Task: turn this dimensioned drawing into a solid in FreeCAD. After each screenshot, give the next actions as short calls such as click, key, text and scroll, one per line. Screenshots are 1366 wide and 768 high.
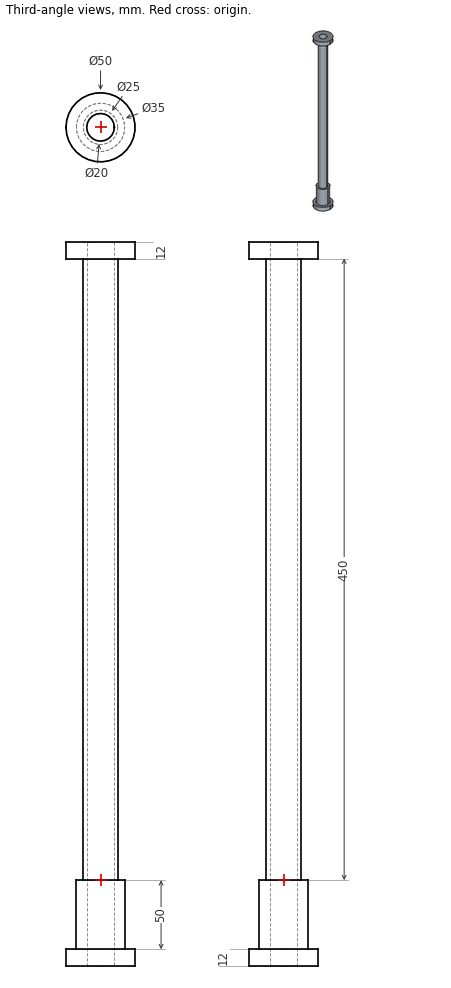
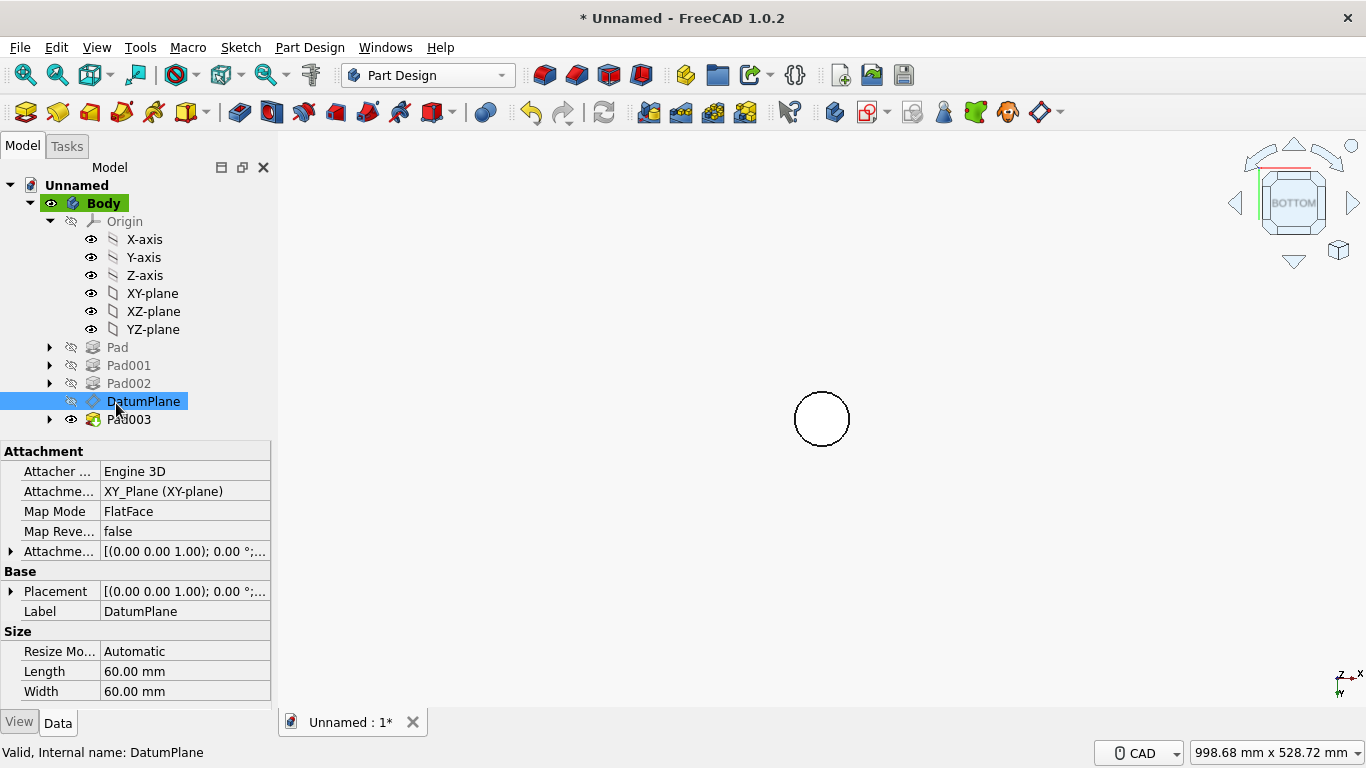
key(0)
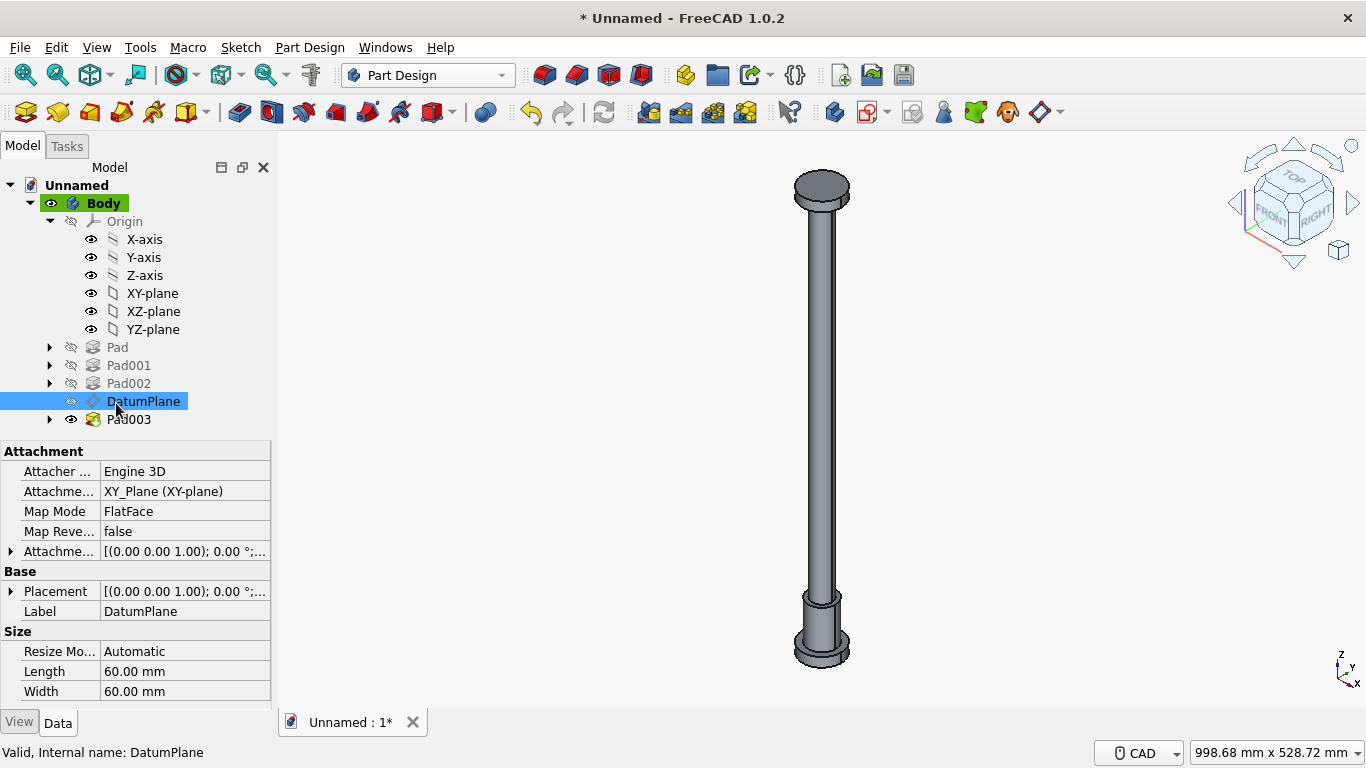
click(822, 185)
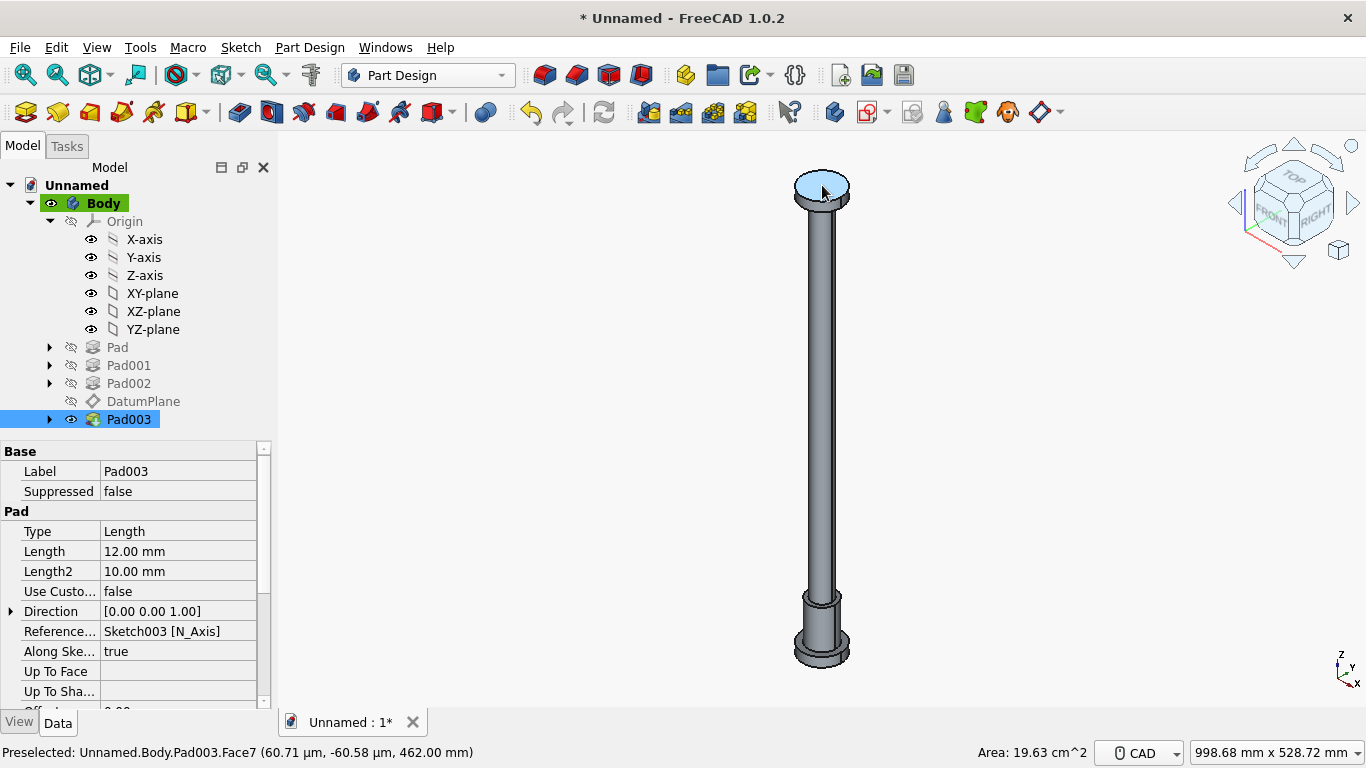
click(868, 112)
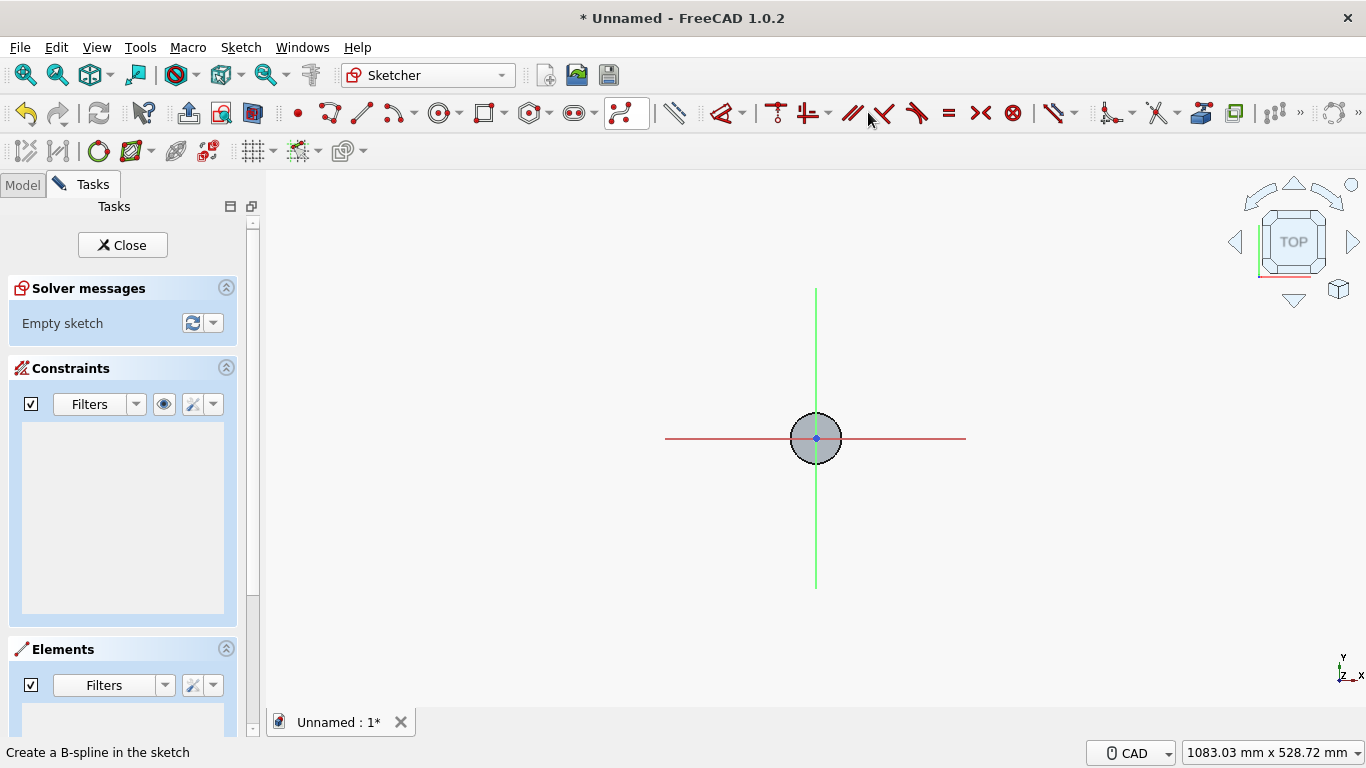
scroll(820, 438, up, 14)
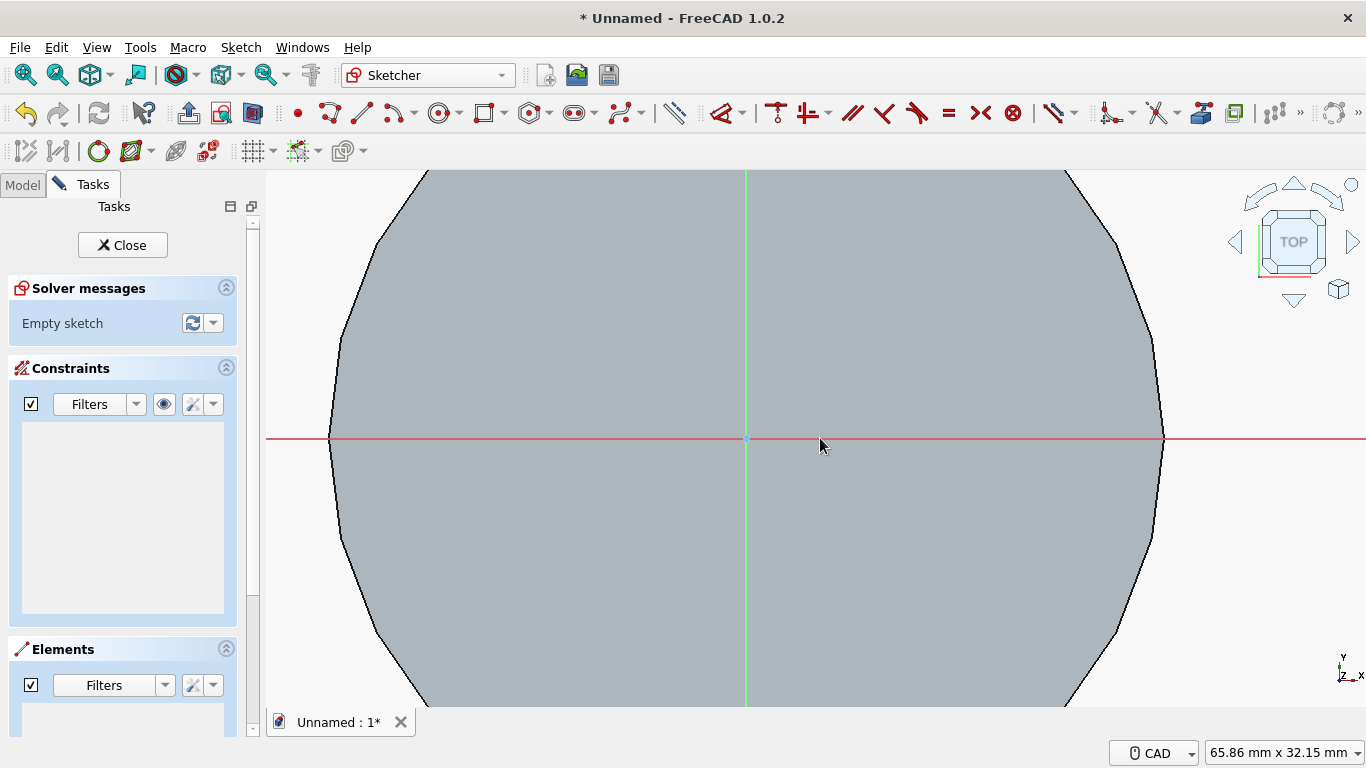
key(g)
key(c)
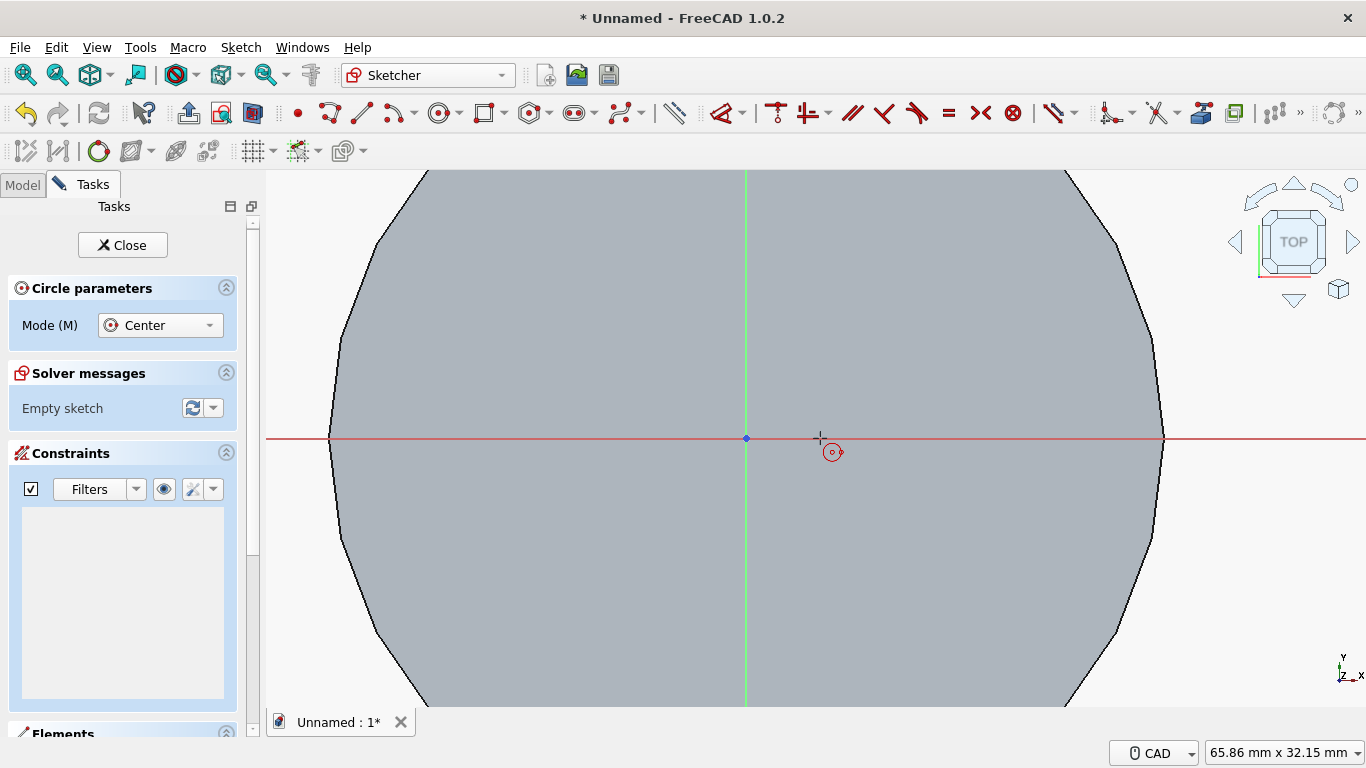
click(746, 438)
click(865, 320)
key(Escape)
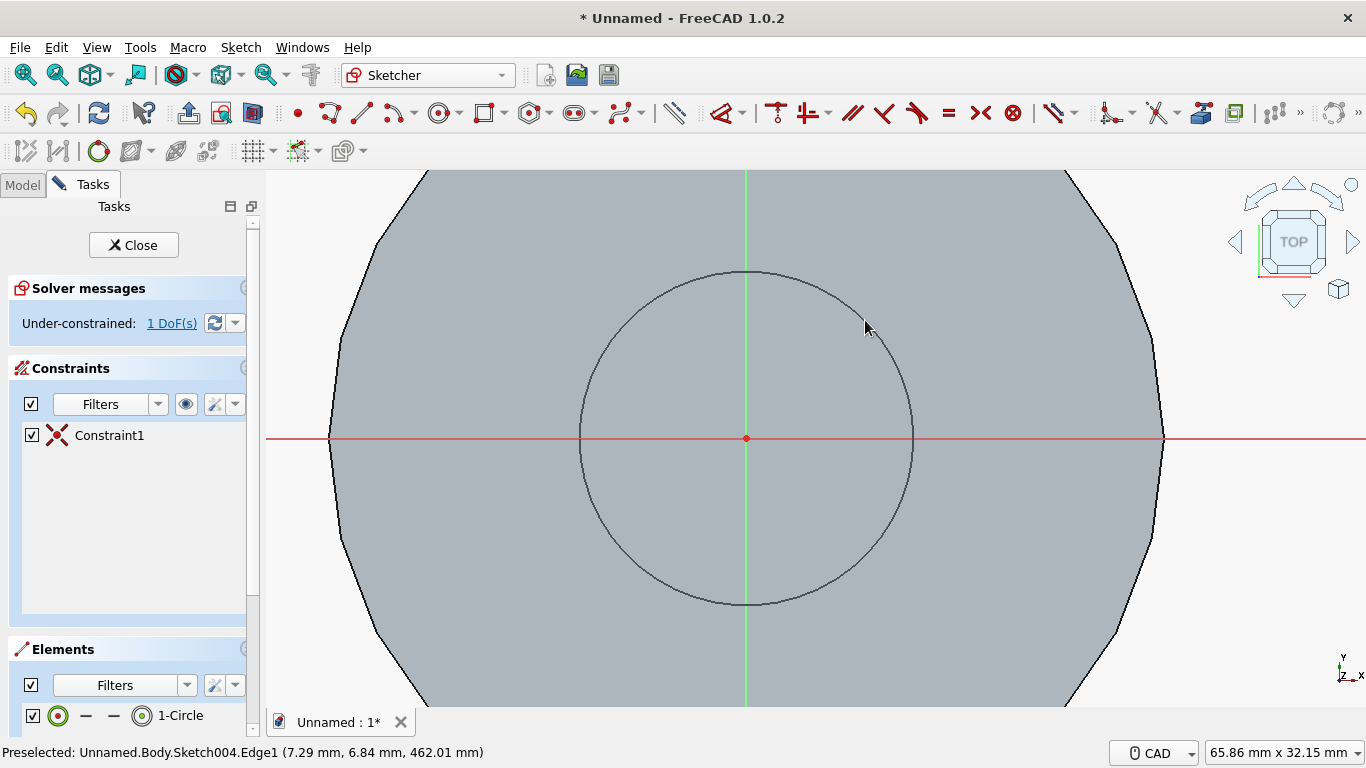
click(722, 114)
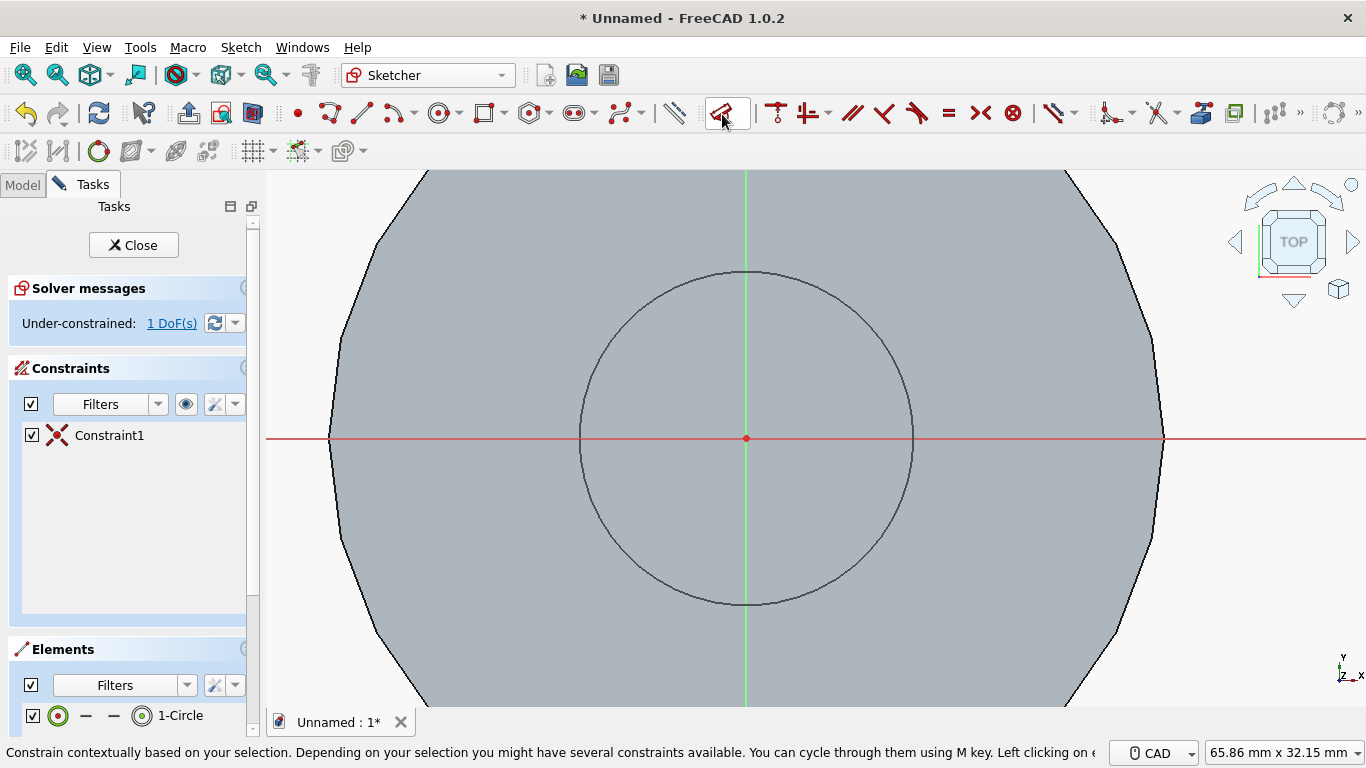
click(864, 320)
click(887, 297)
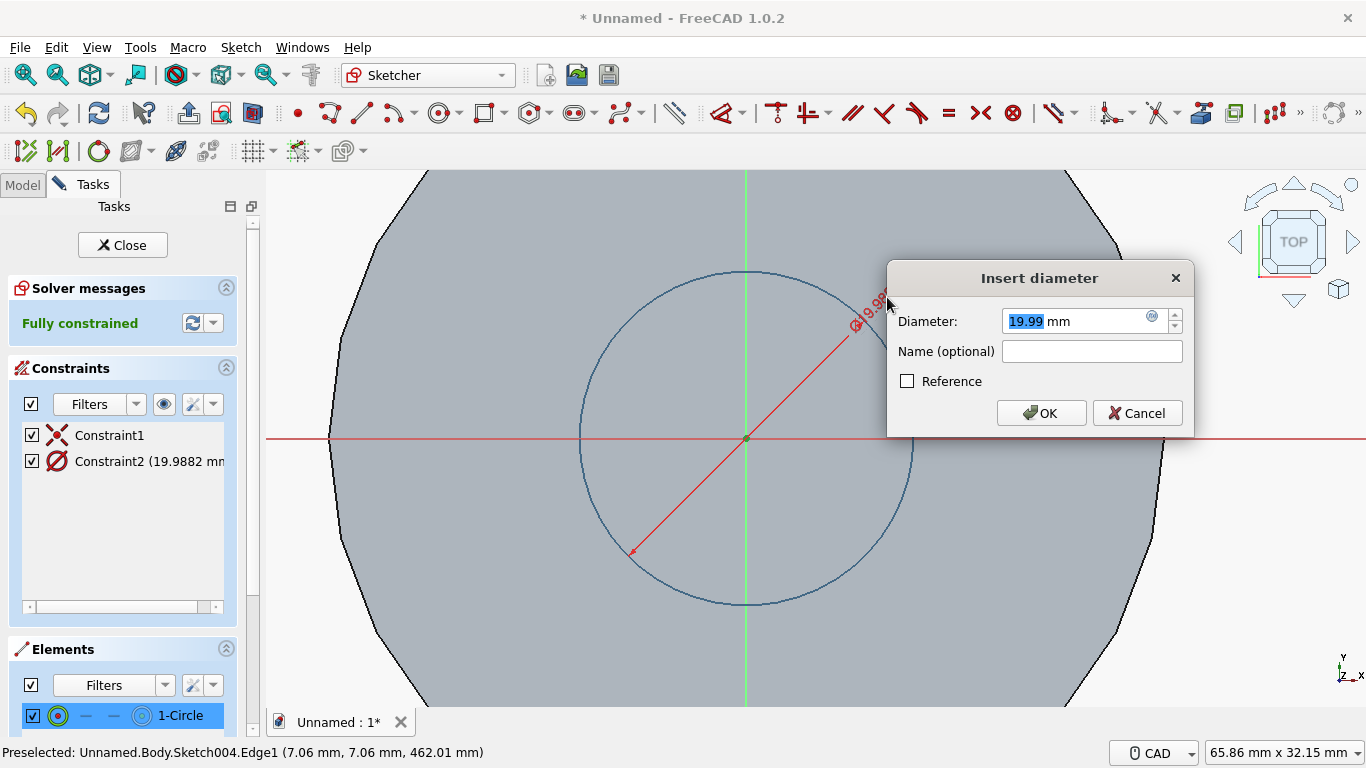
text(20)
key(Return)
key(Escape)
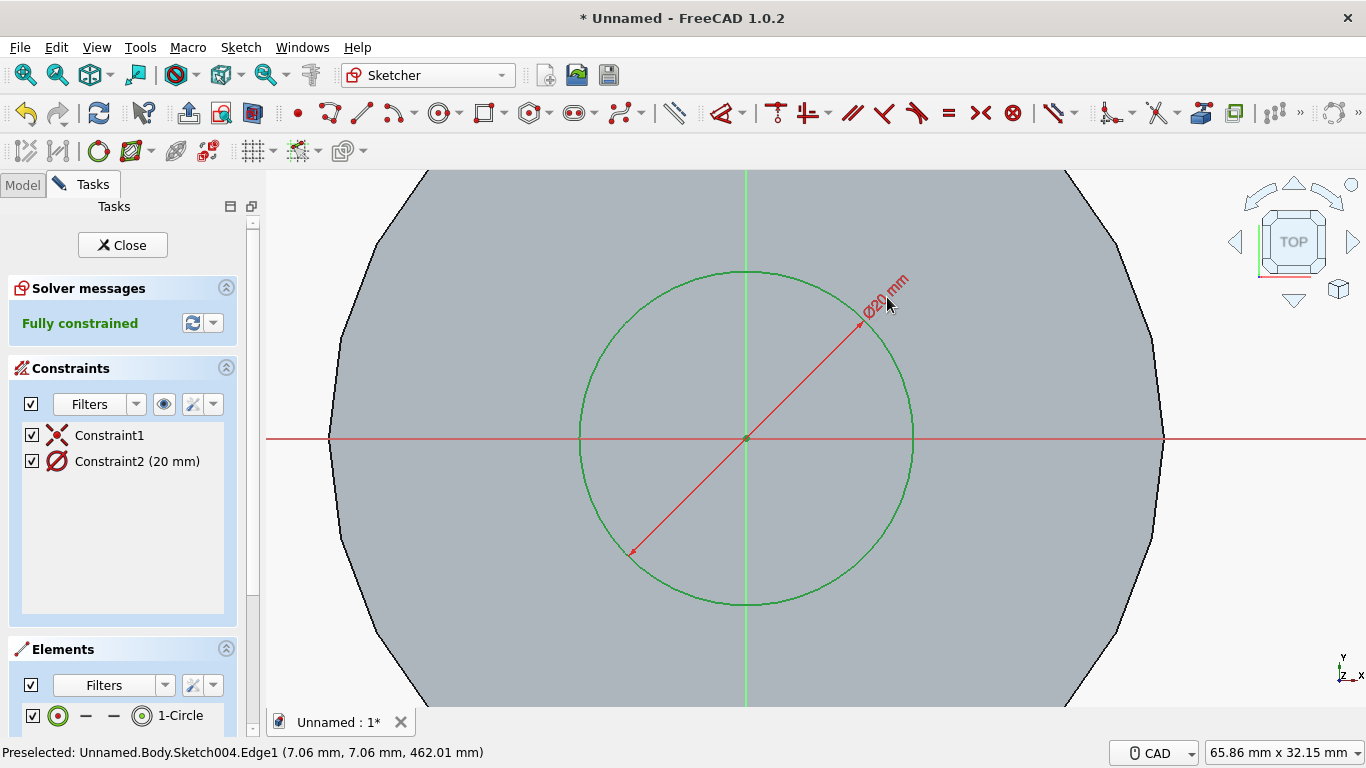
click(123, 245)